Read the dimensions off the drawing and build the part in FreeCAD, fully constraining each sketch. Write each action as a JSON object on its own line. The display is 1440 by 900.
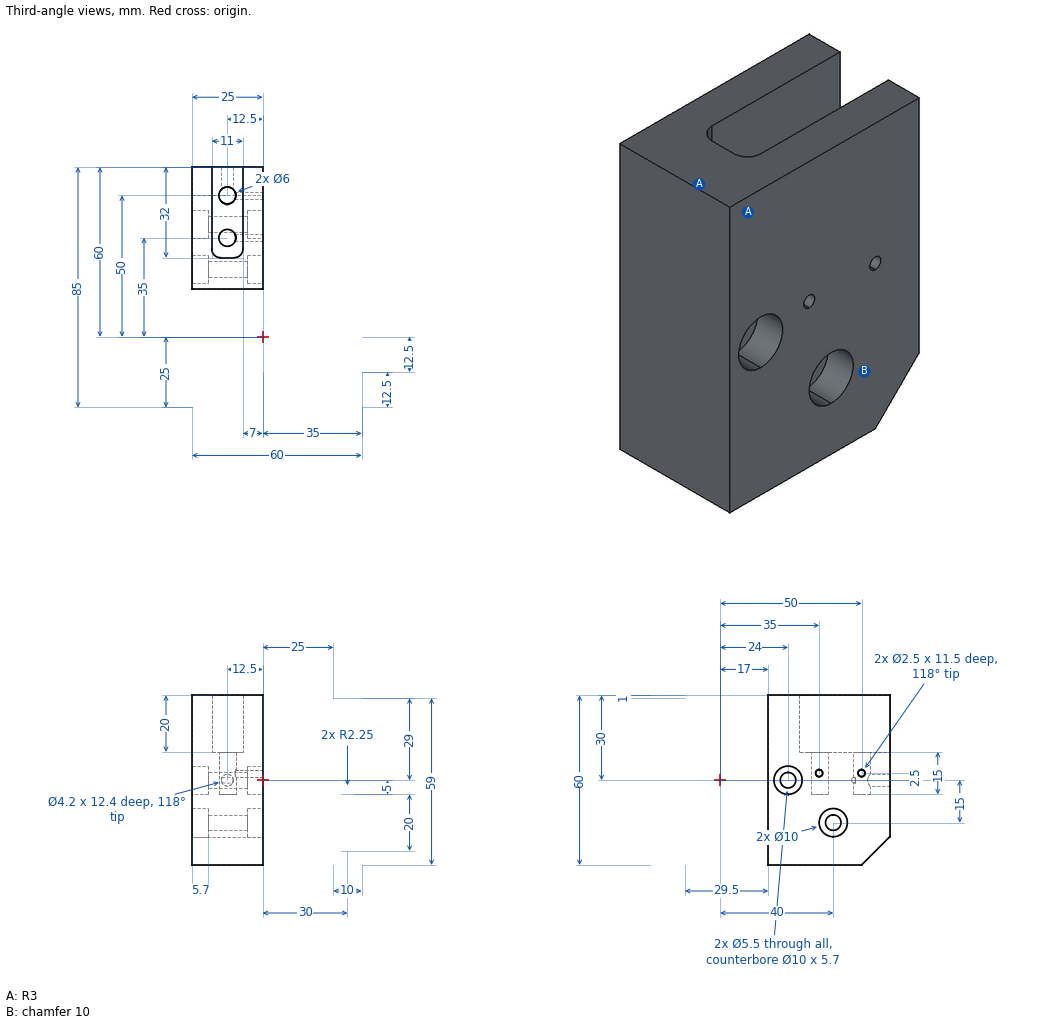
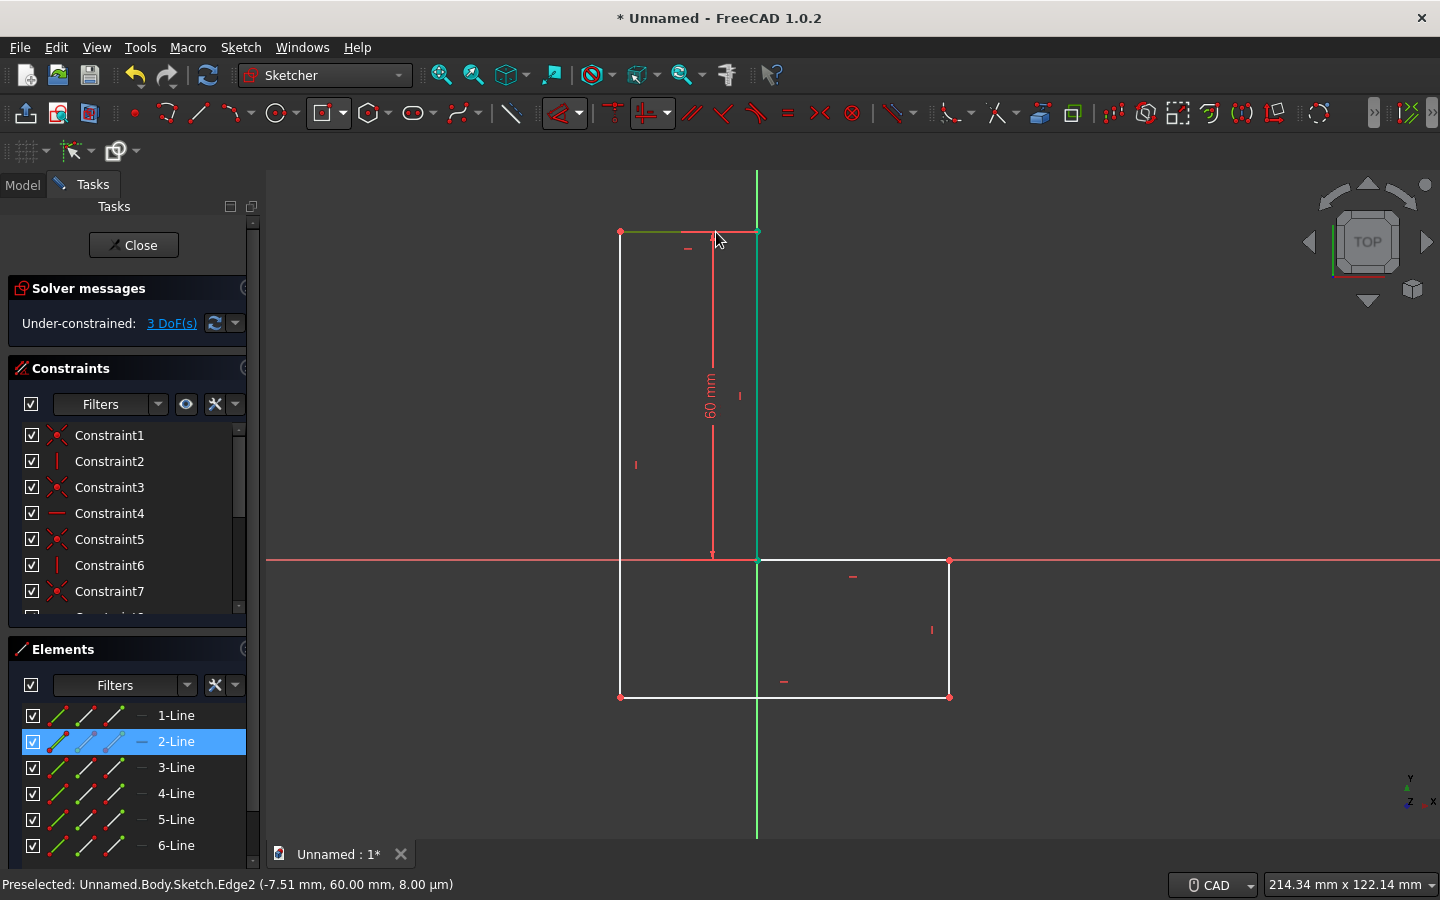
{"action": "left_click", "coordinate": [582, 114]}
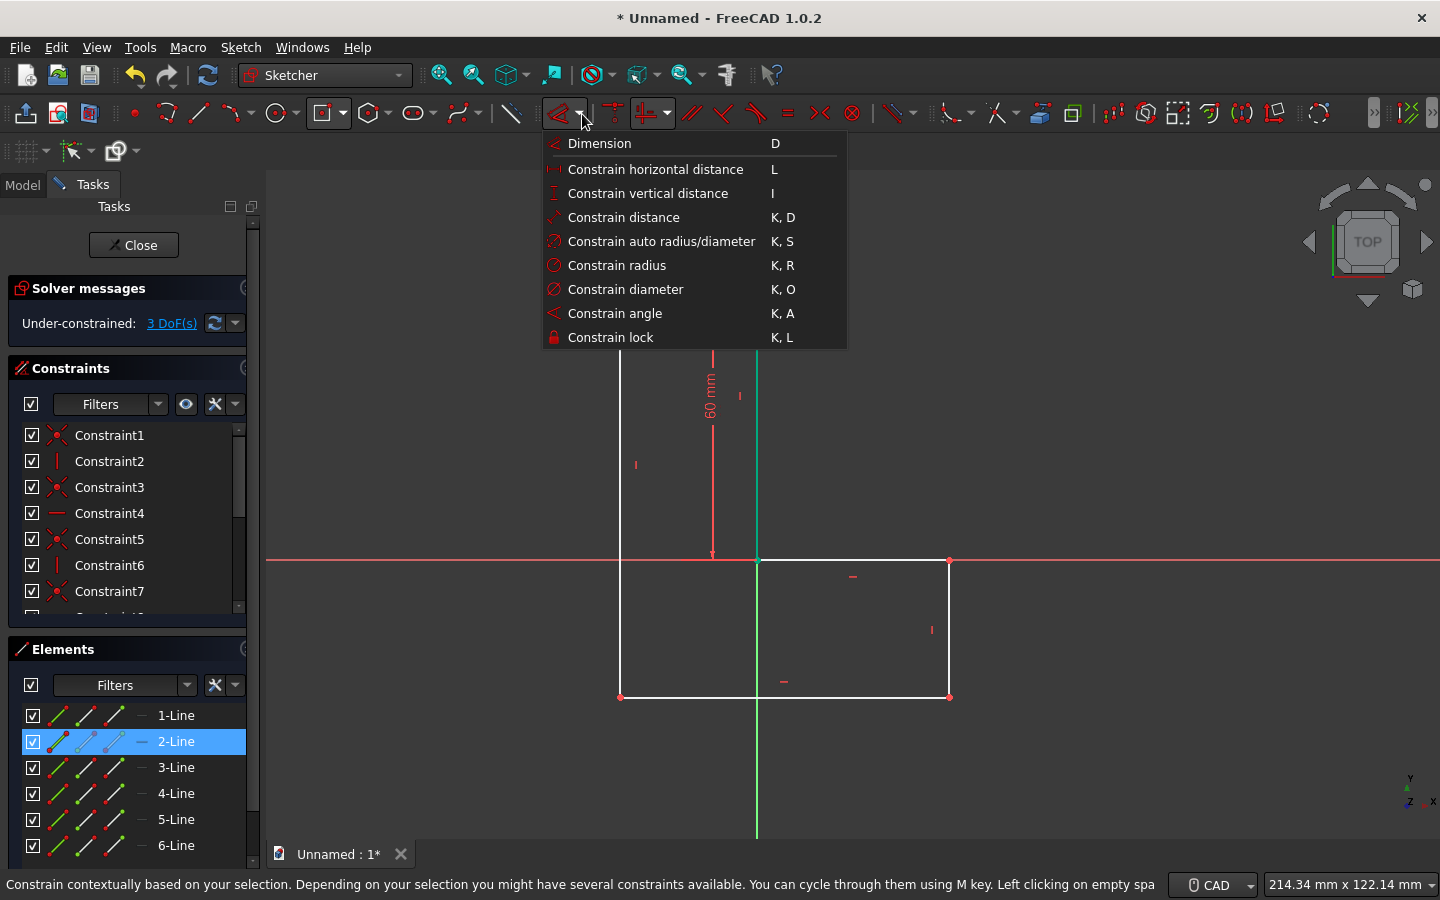
{"action": "left_click", "coordinate": [695, 169]}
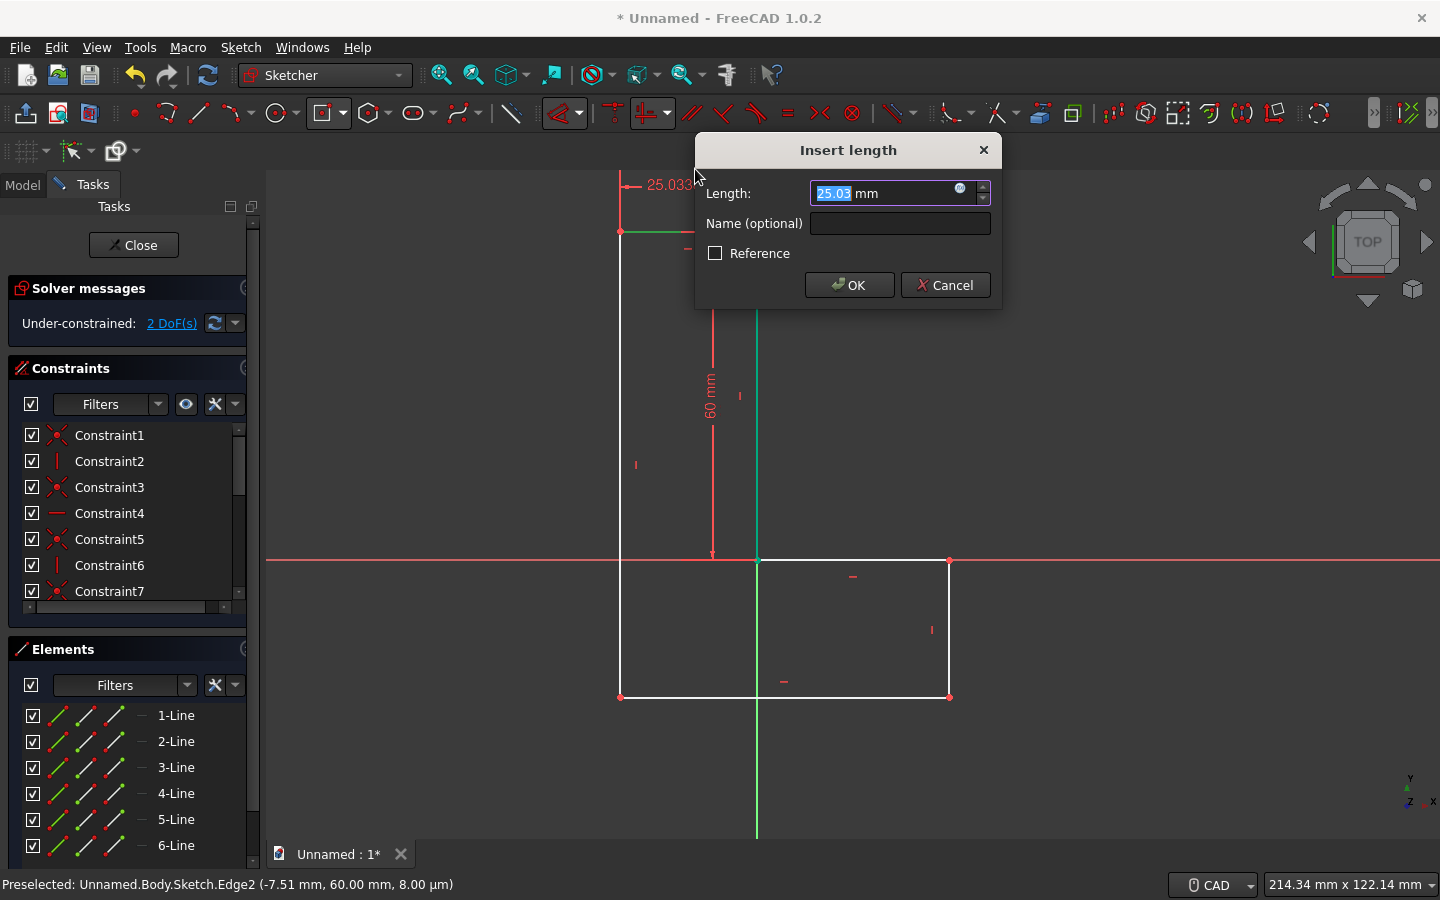
{"action": "type", "text": "25"}
{"action": "key", "text": "Return"}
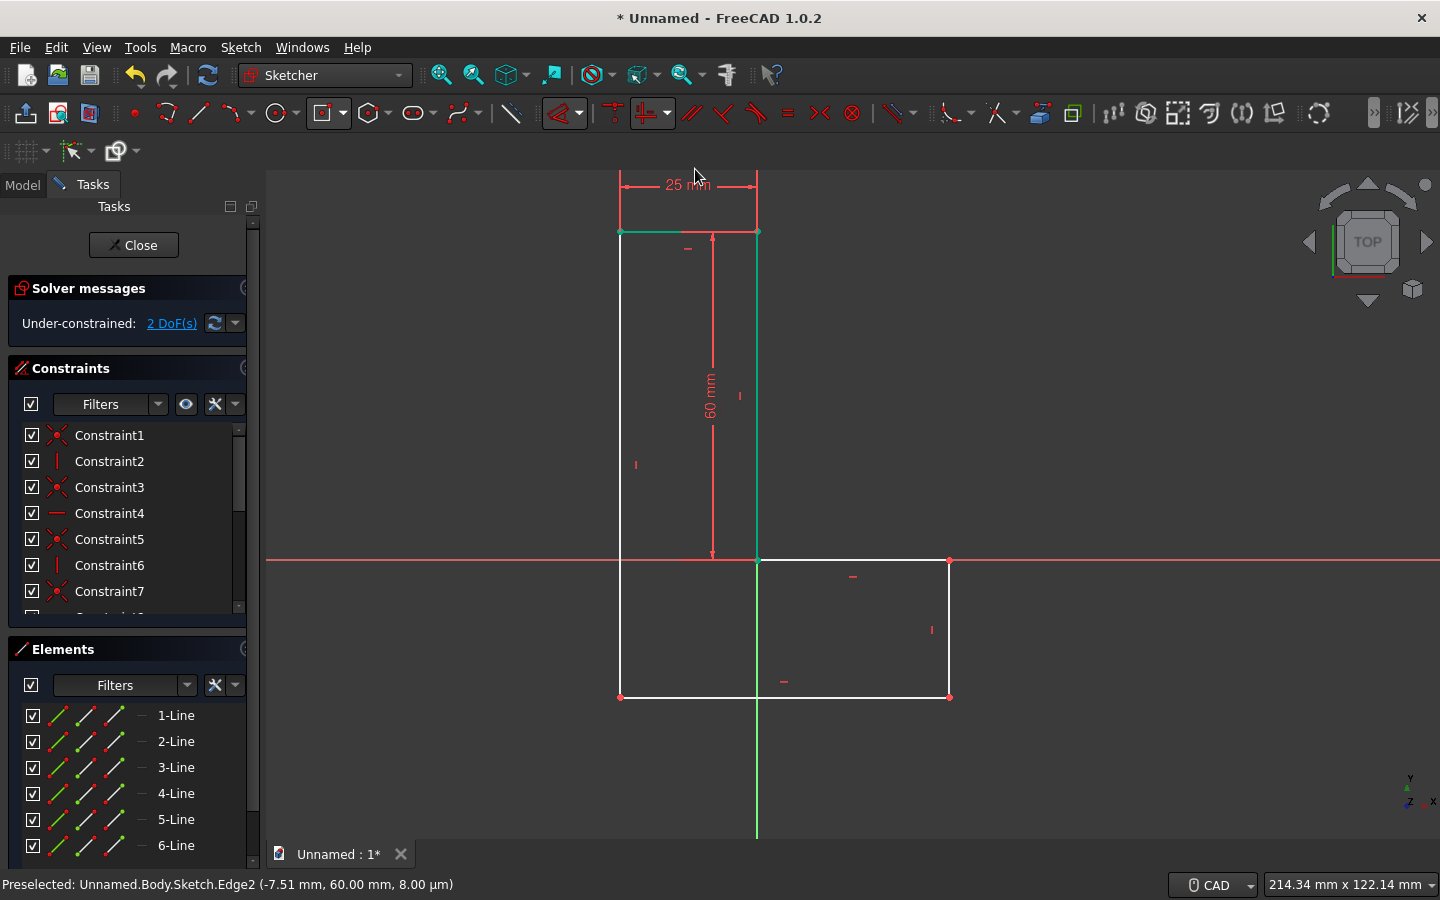
{"action": "left_click", "coordinate": [620, 372]}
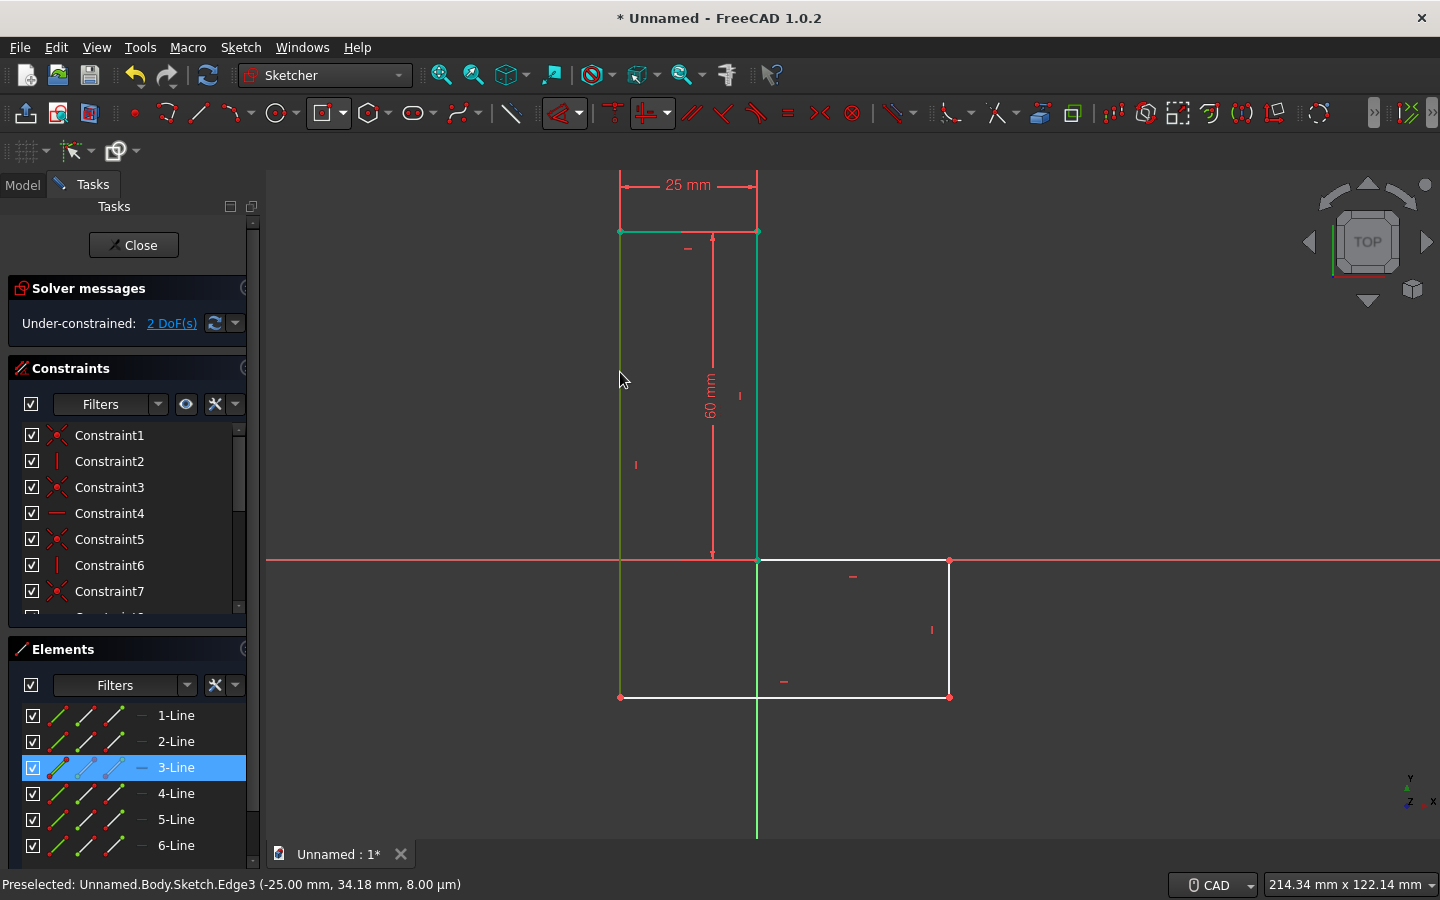
{"action": "left_click", "coordinate": [582, 114]}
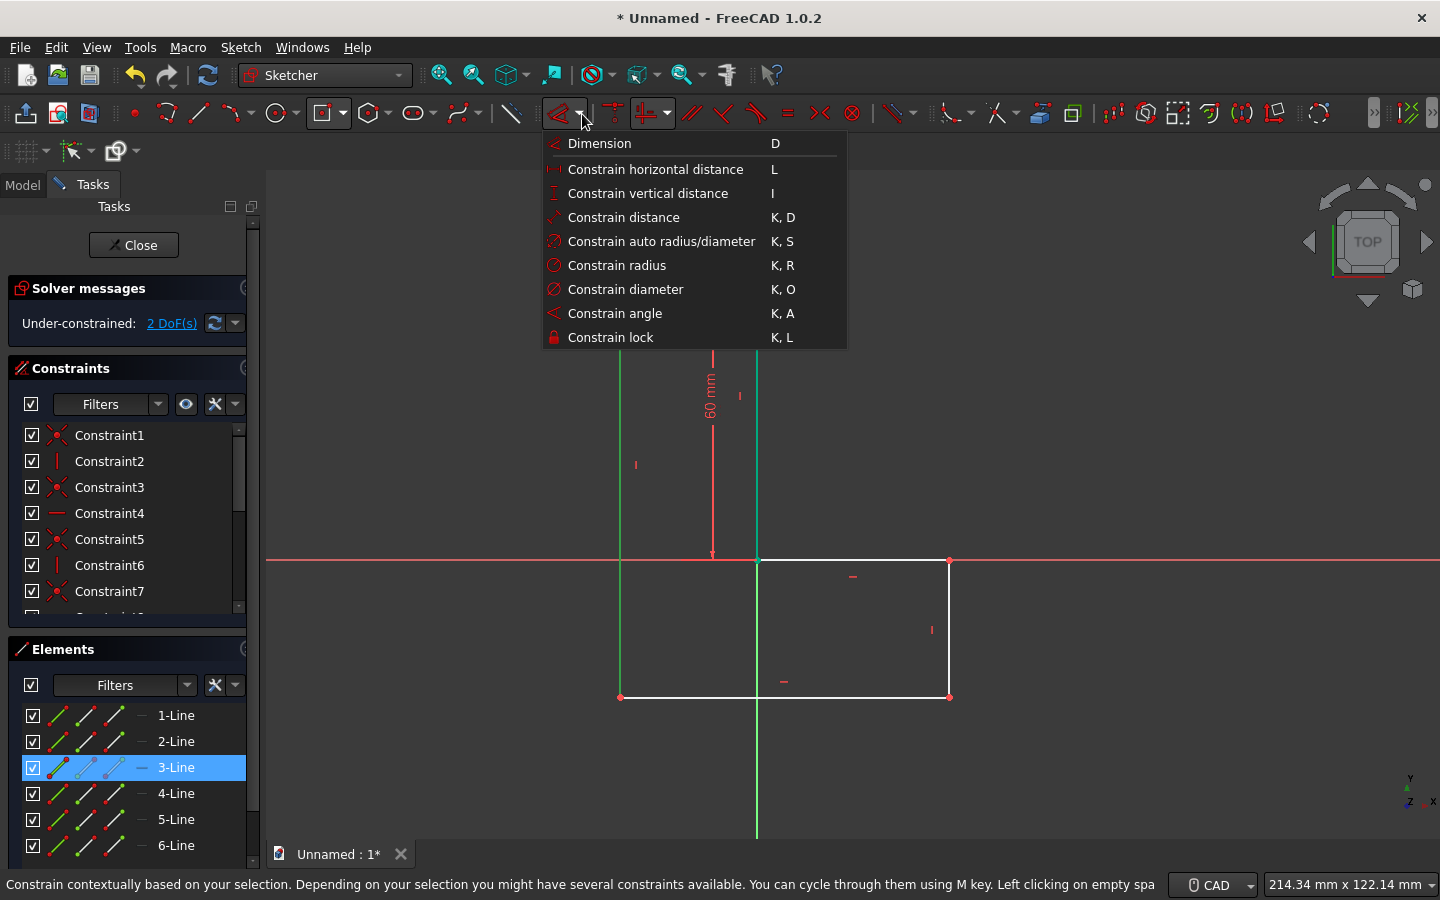
{"action": "left_click", "coordinate": [695, 193]}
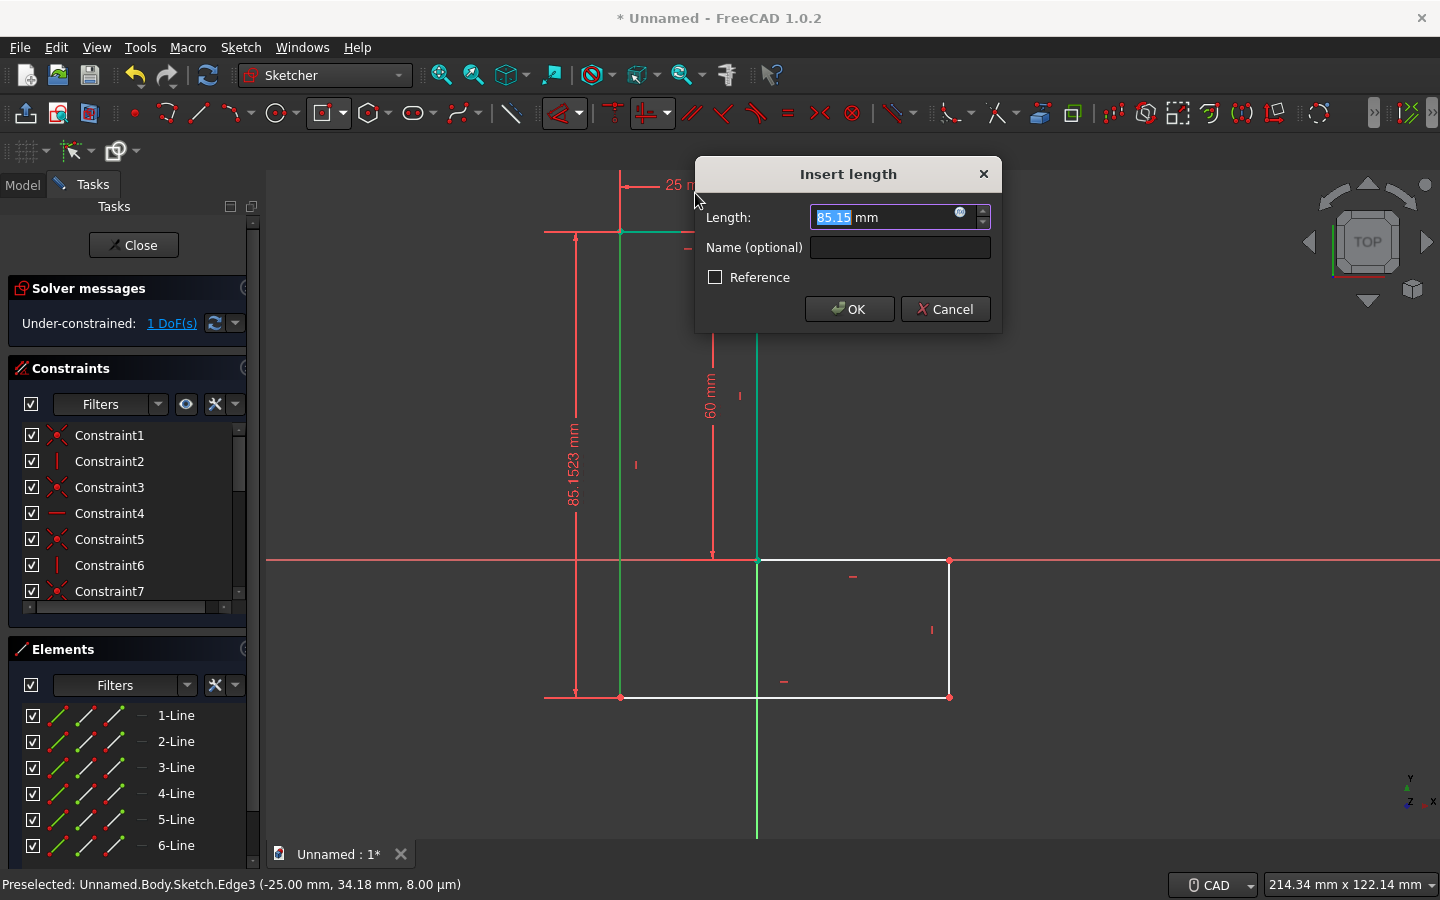
{"action": "type", "text": "85"}
{"action": "key", "text": "Return"}